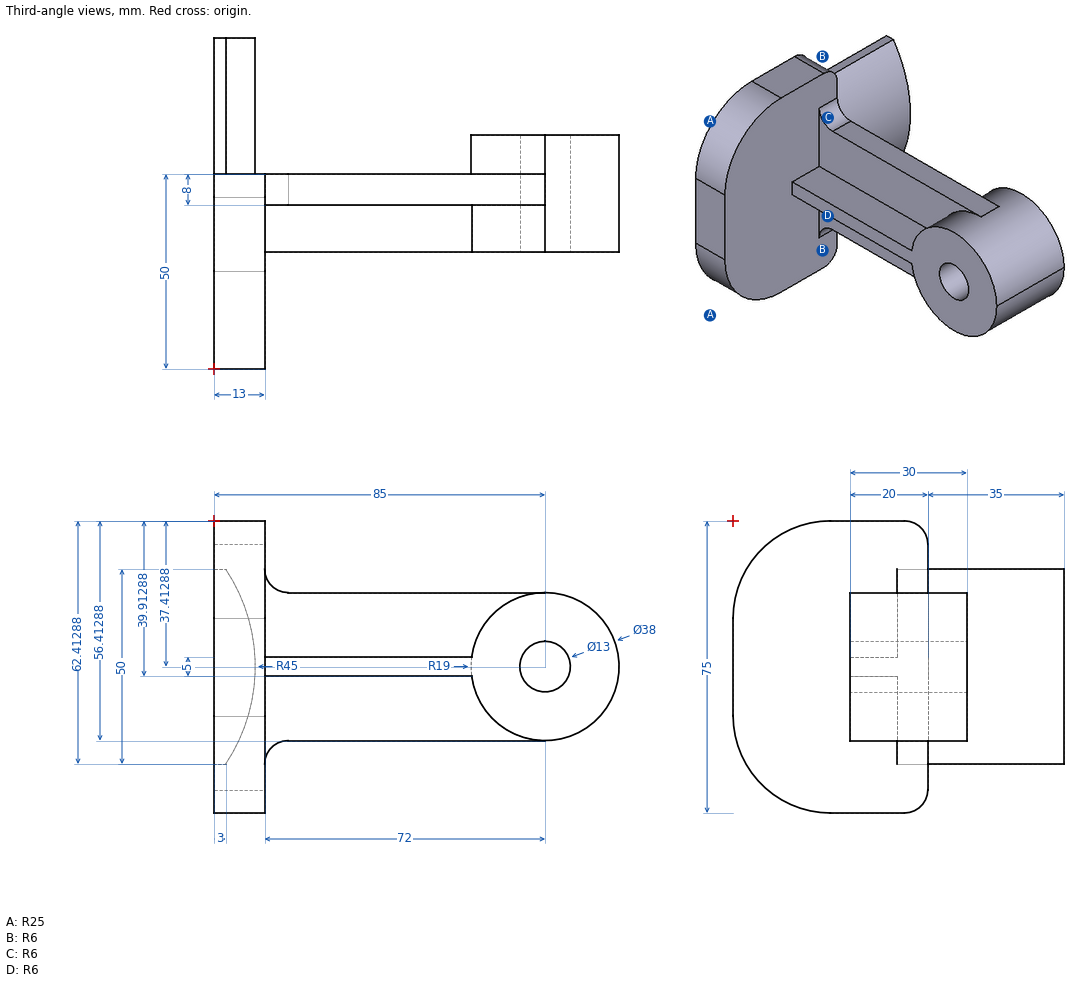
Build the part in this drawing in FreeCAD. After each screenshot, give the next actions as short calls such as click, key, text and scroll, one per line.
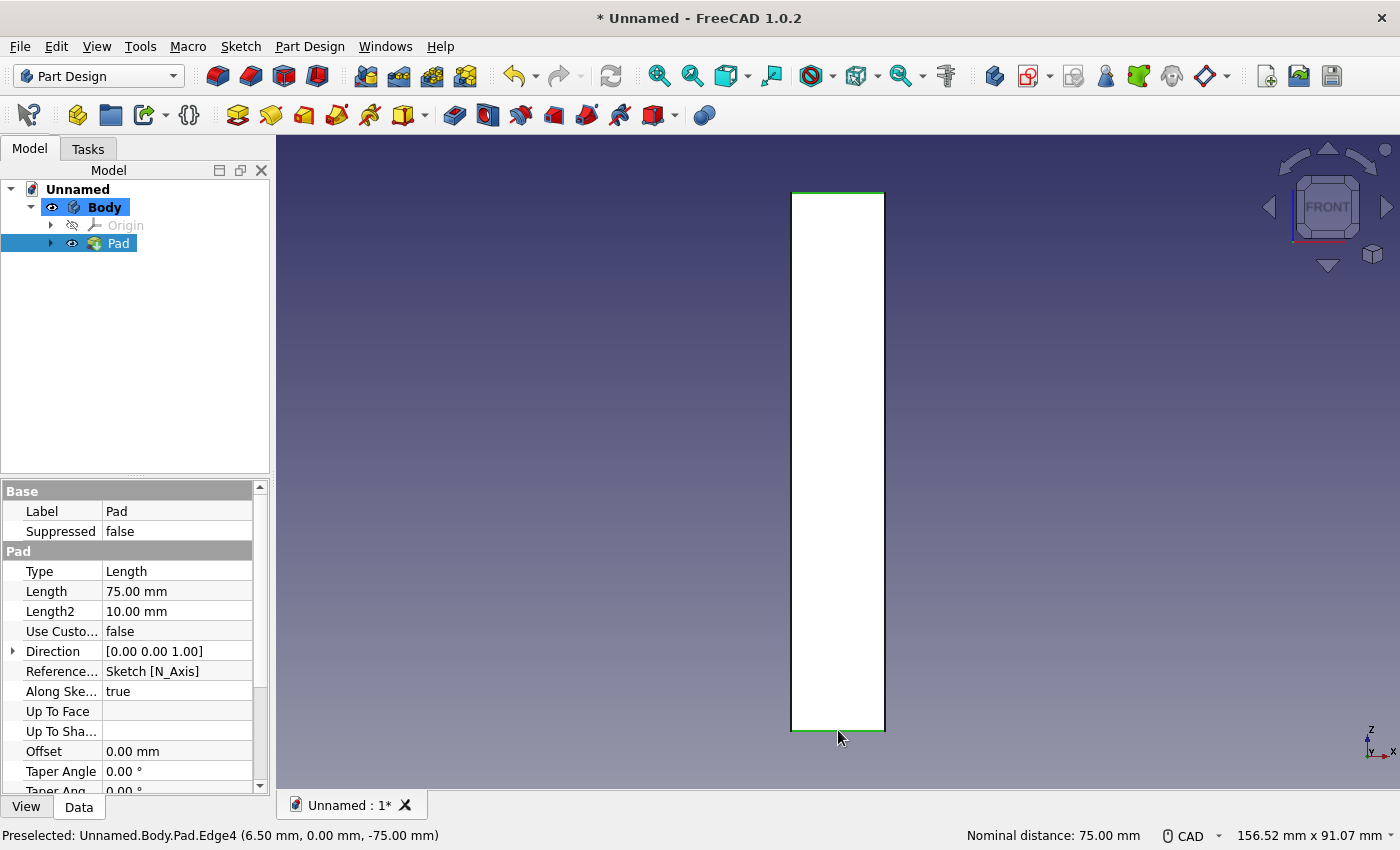
click(218, 76)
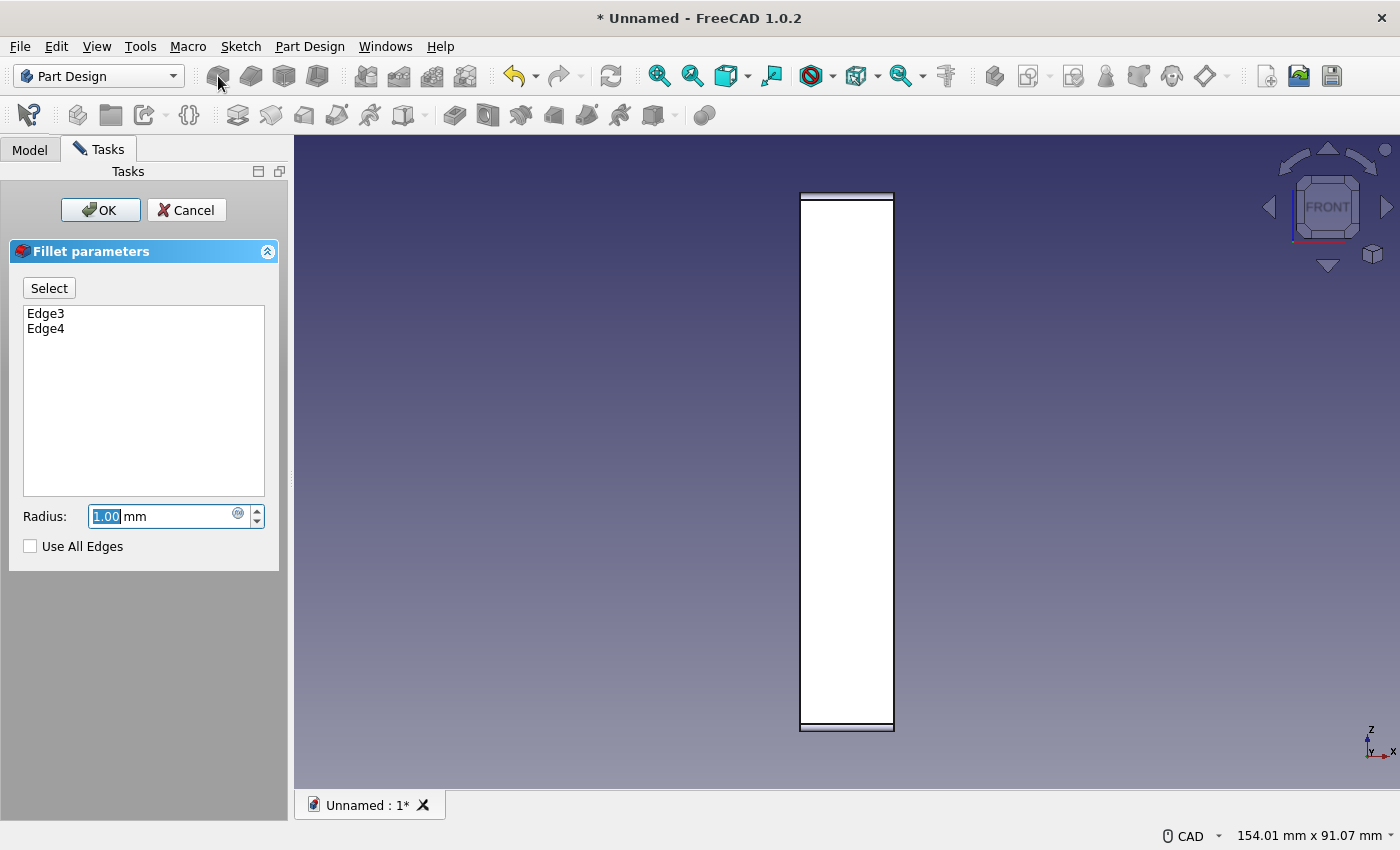
text(25)
key(Tab)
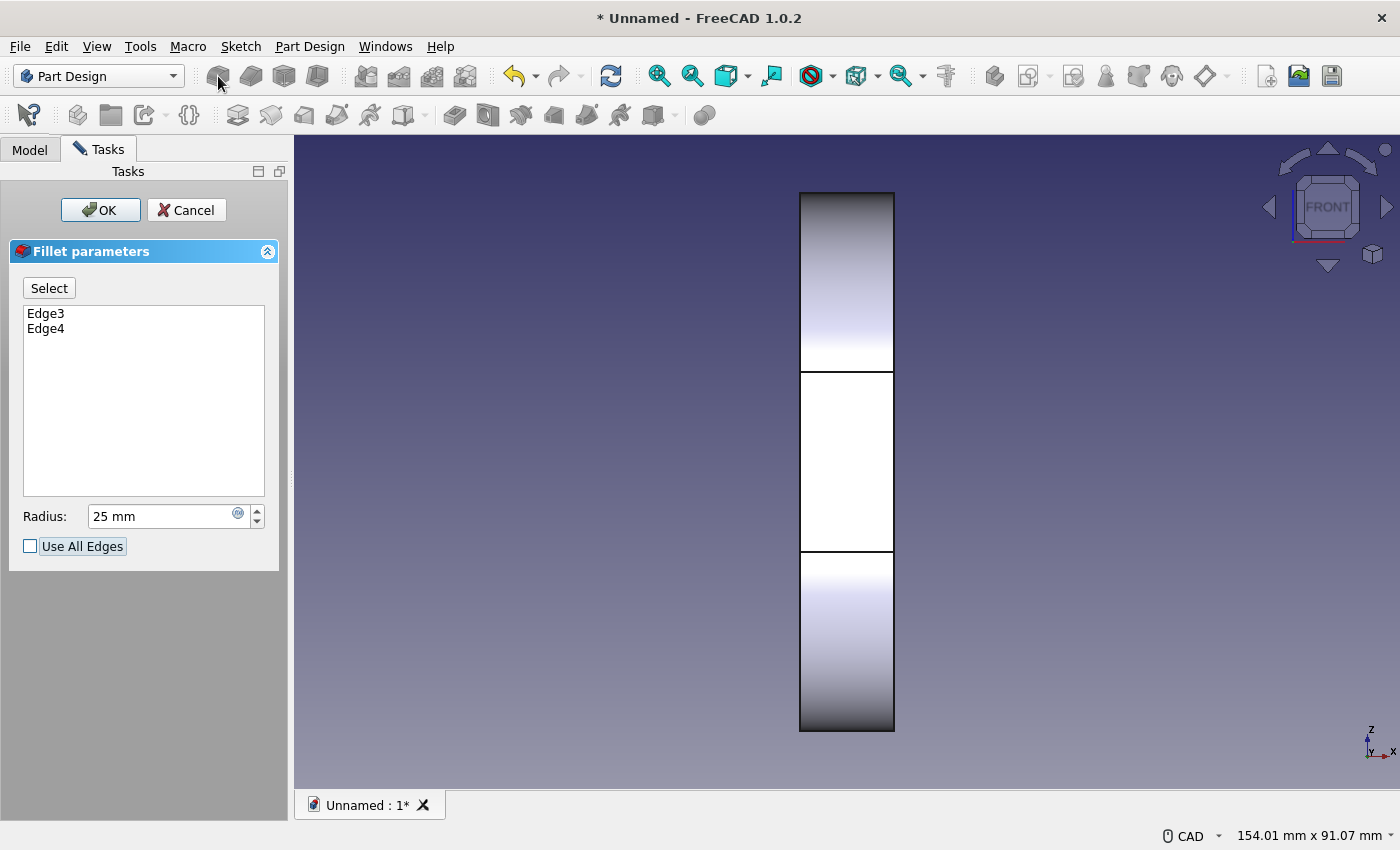
click(101, 210)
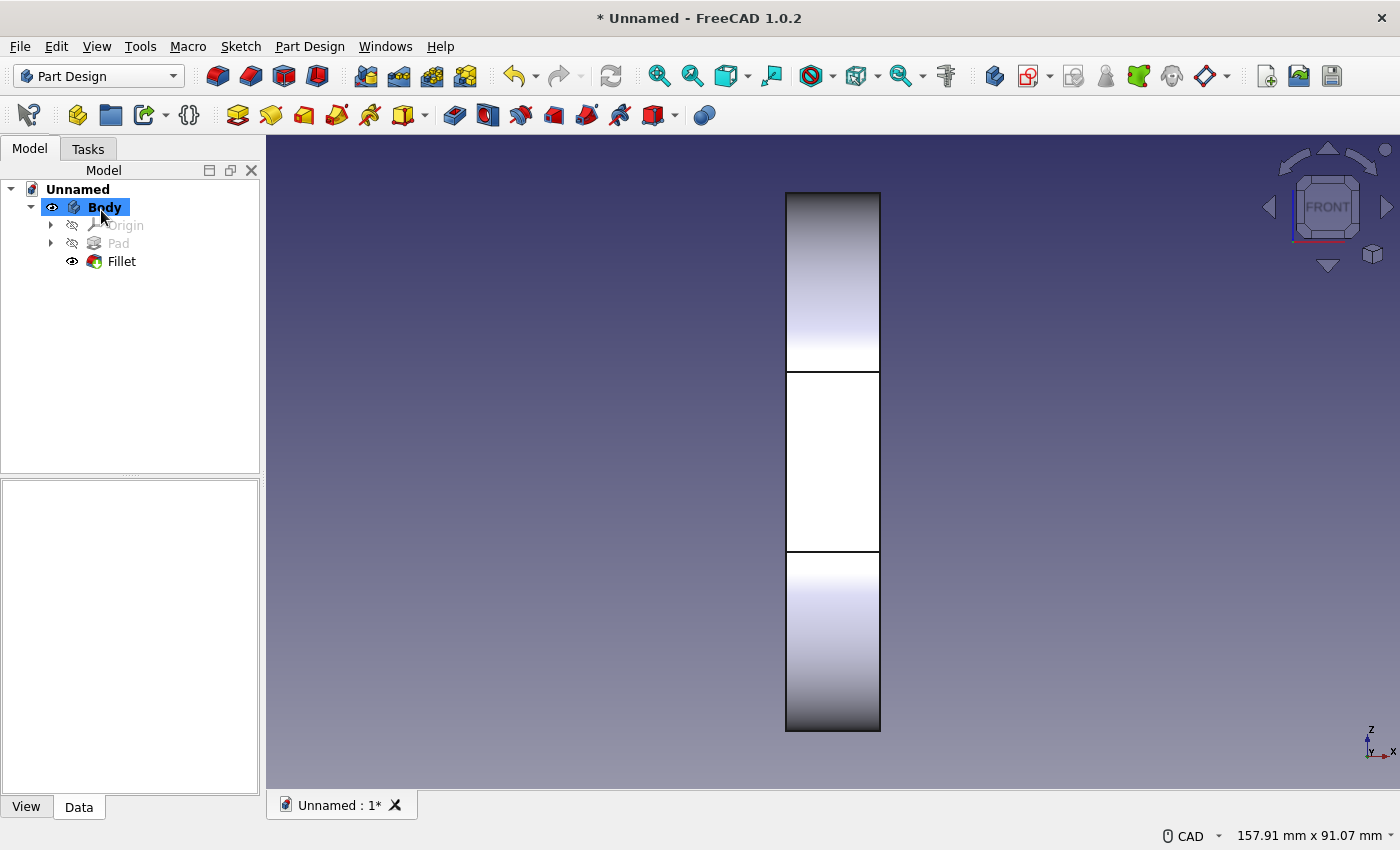
key(0)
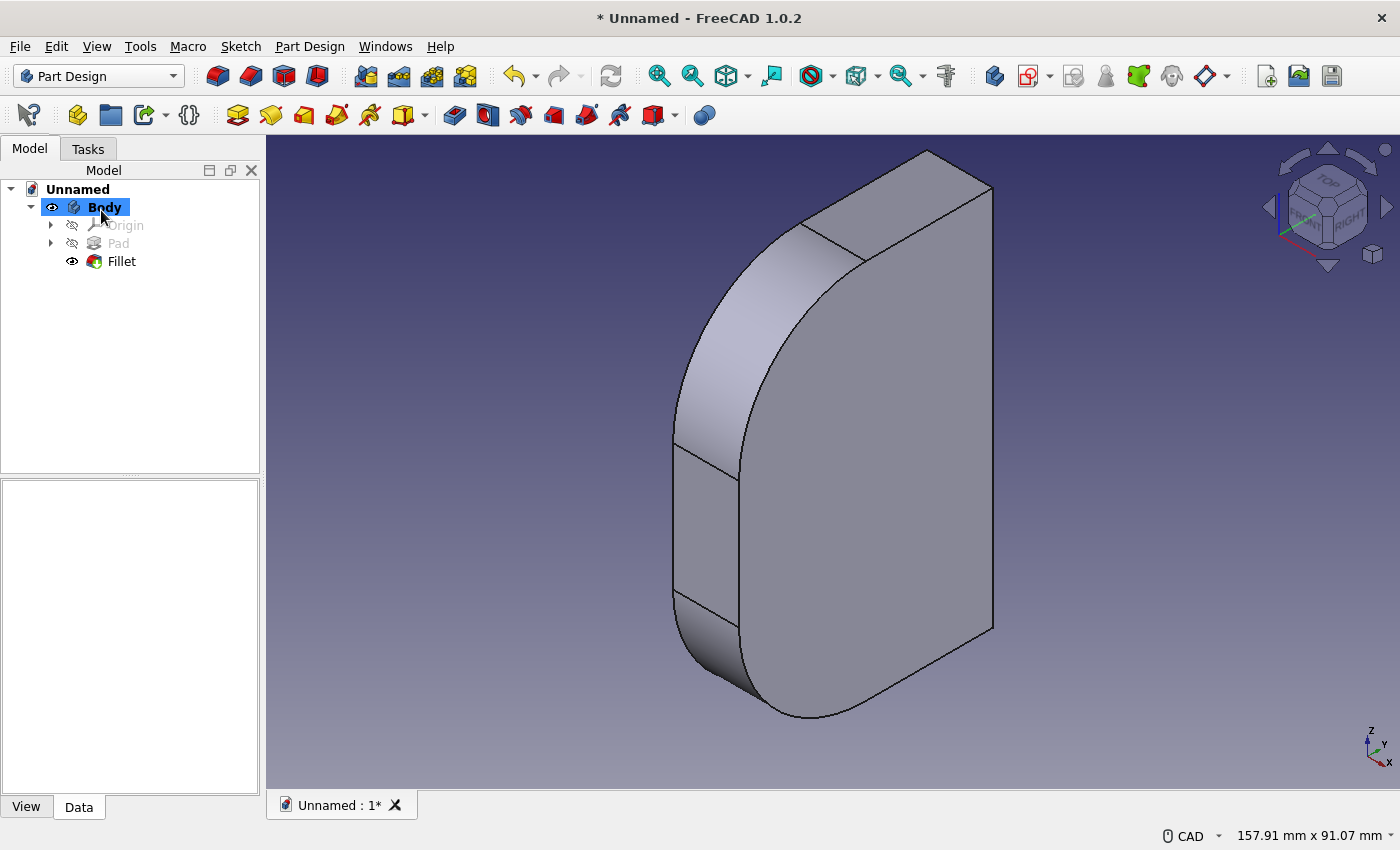
key(2)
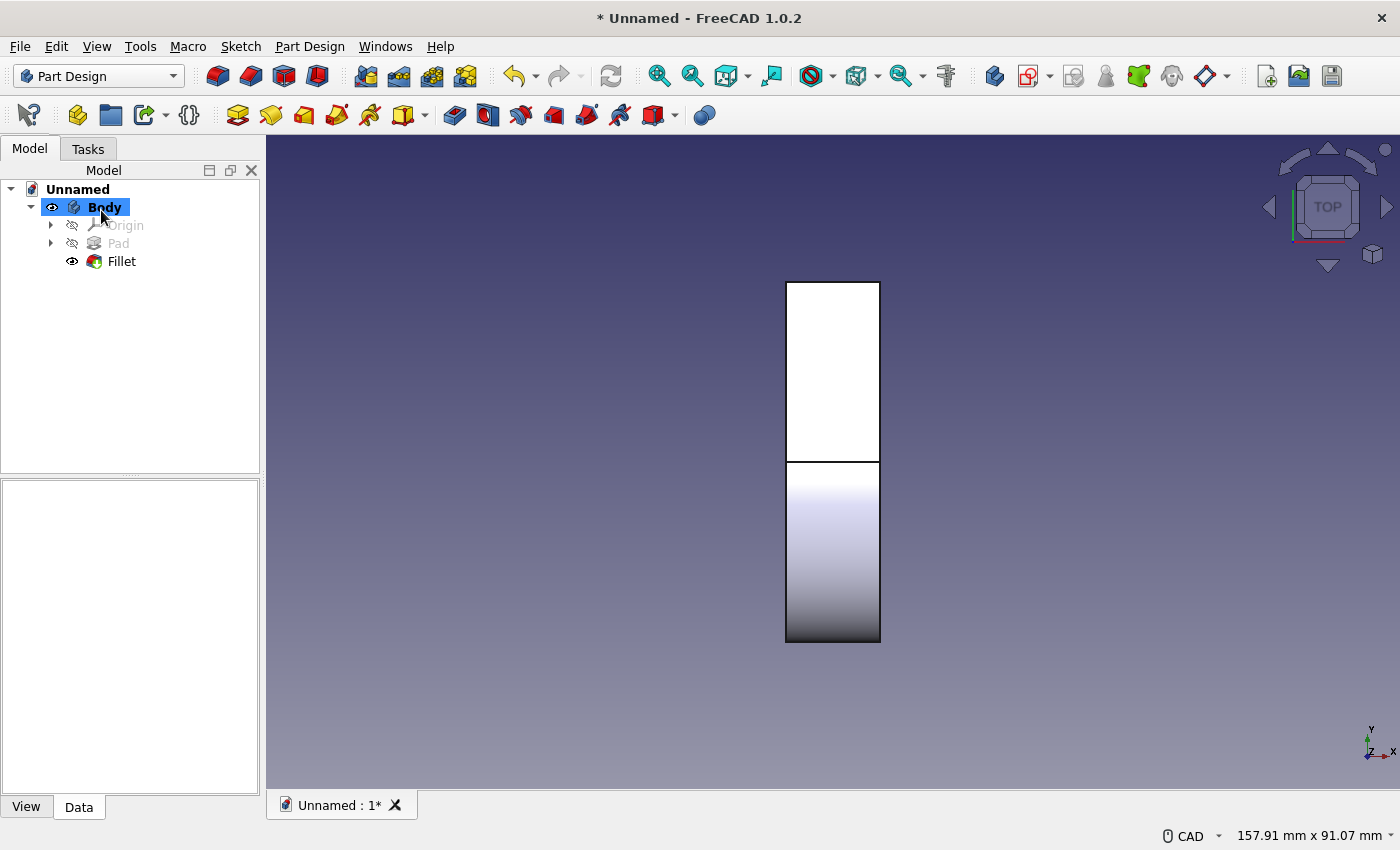
key(1)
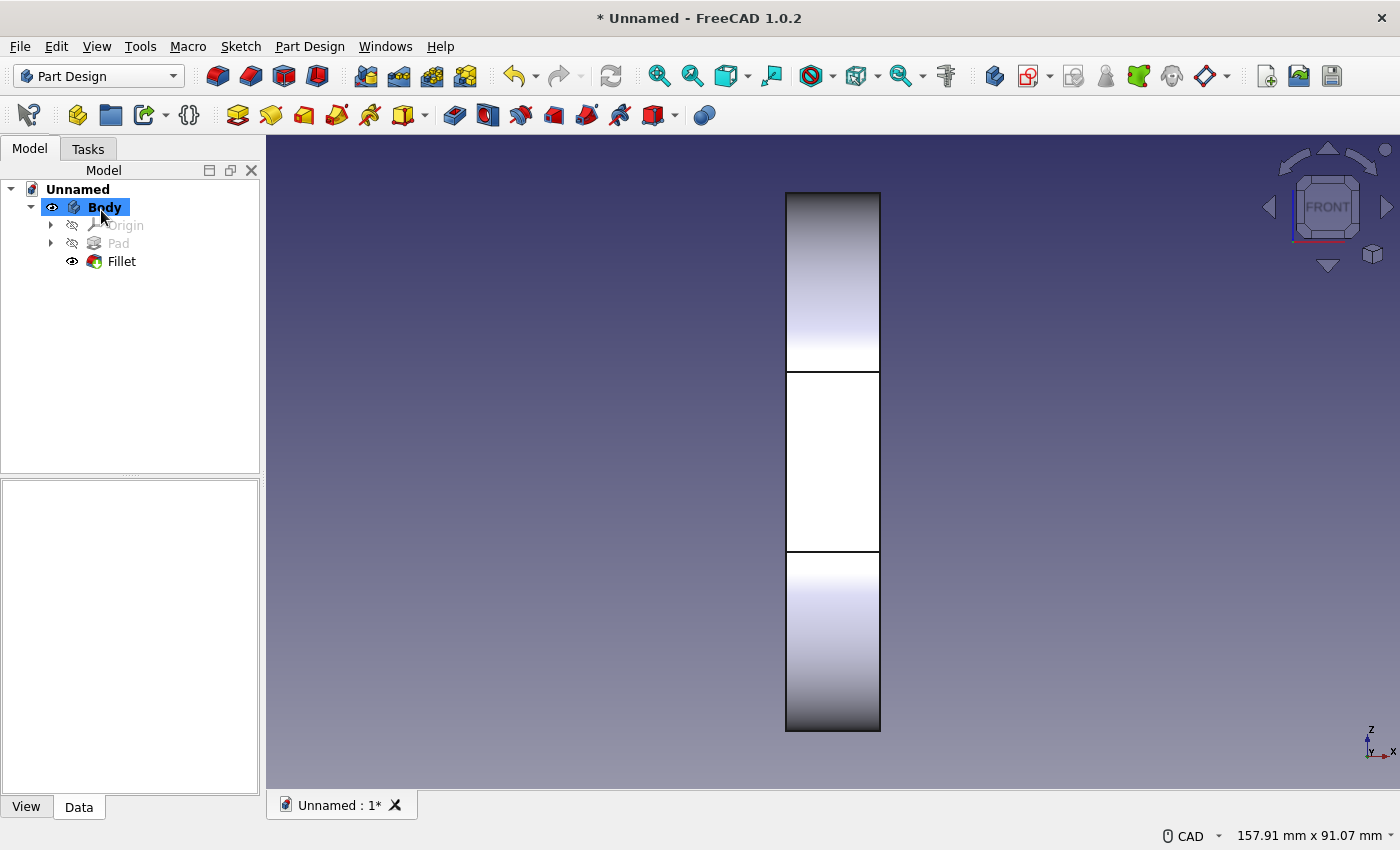
key(3)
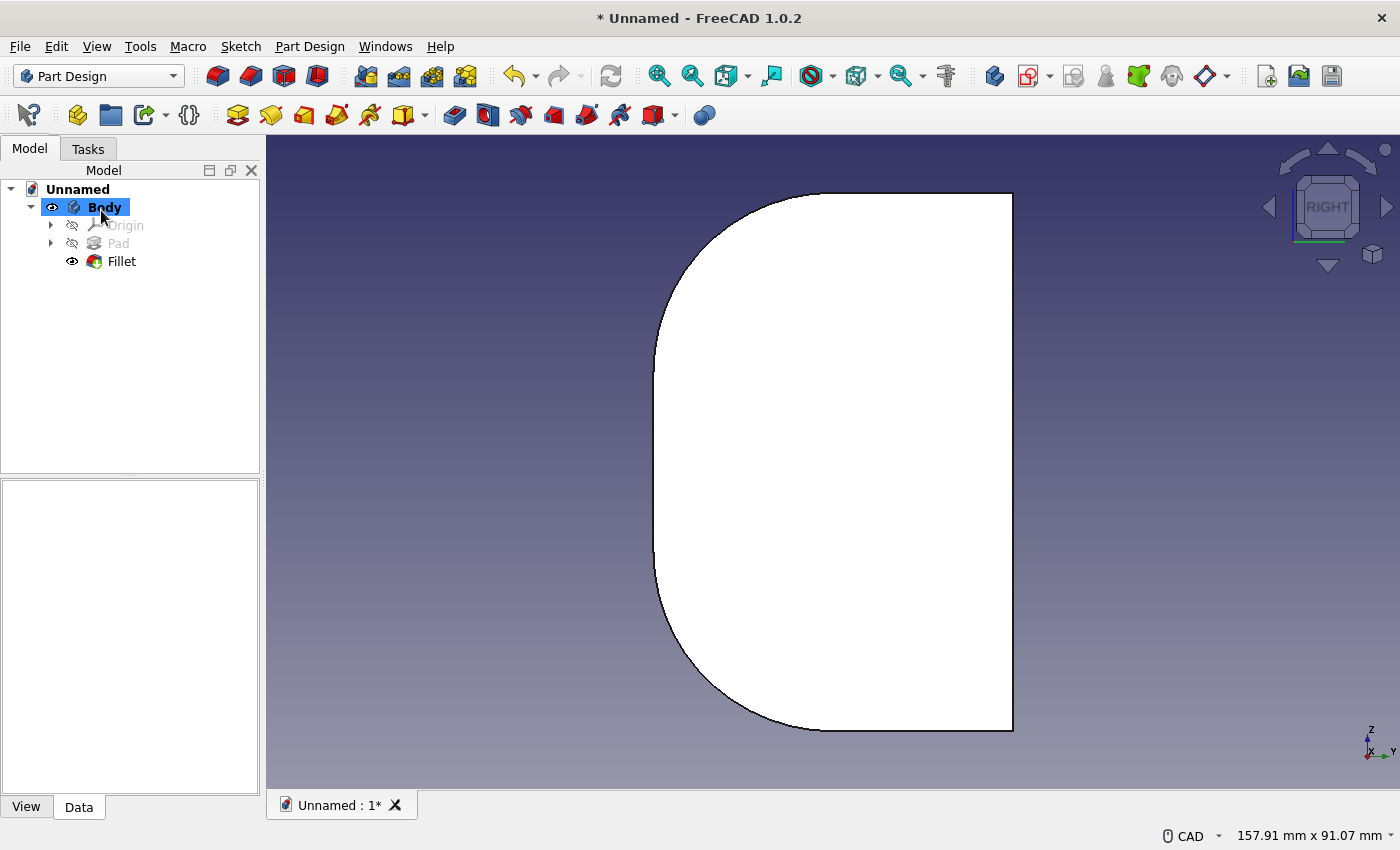
key(5)